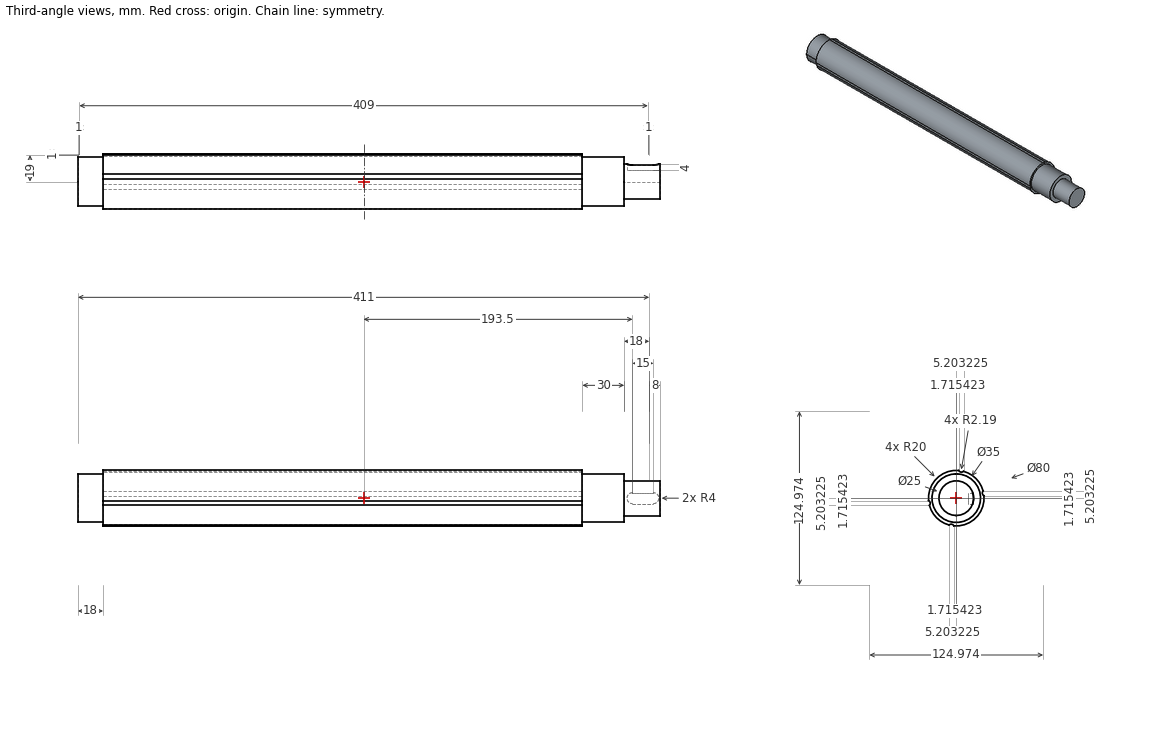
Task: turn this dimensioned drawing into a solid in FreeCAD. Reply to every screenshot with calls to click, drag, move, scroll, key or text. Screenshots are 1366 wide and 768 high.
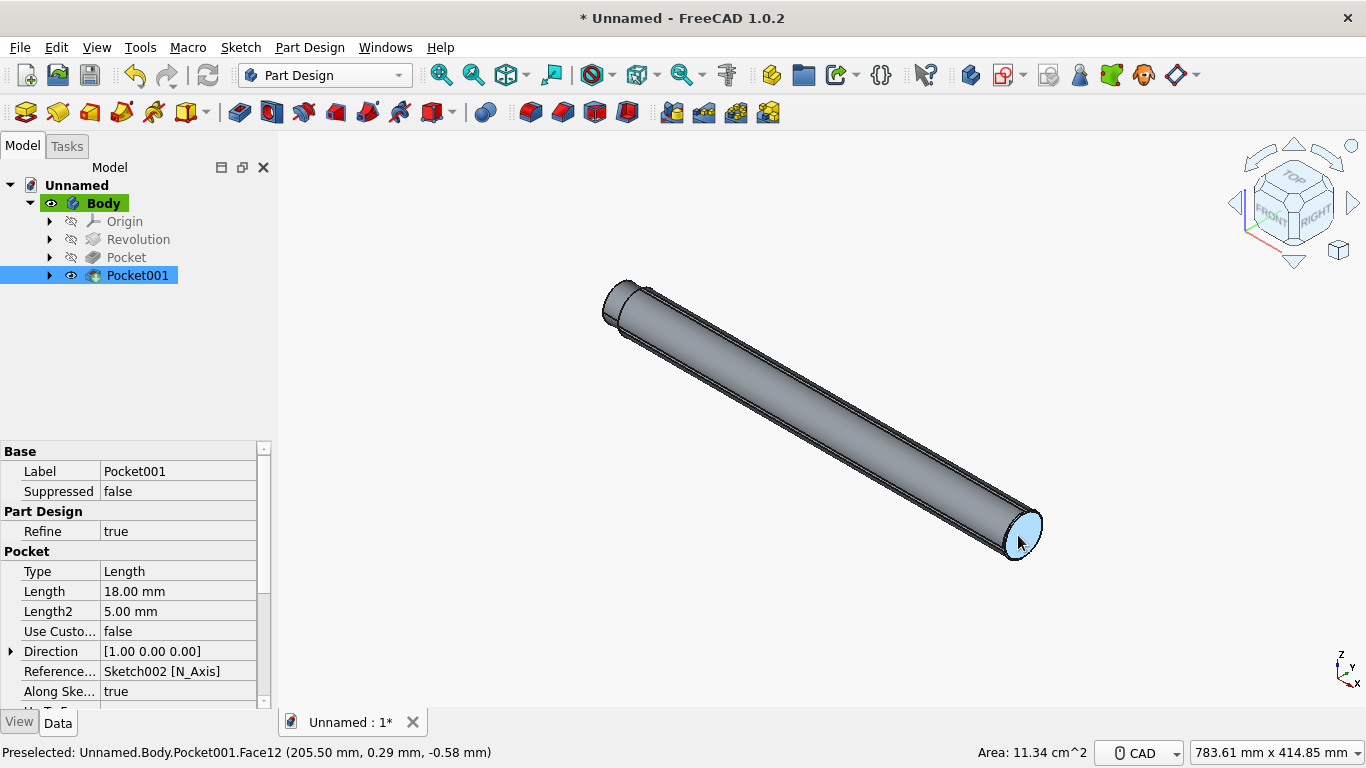
click(1004, 76)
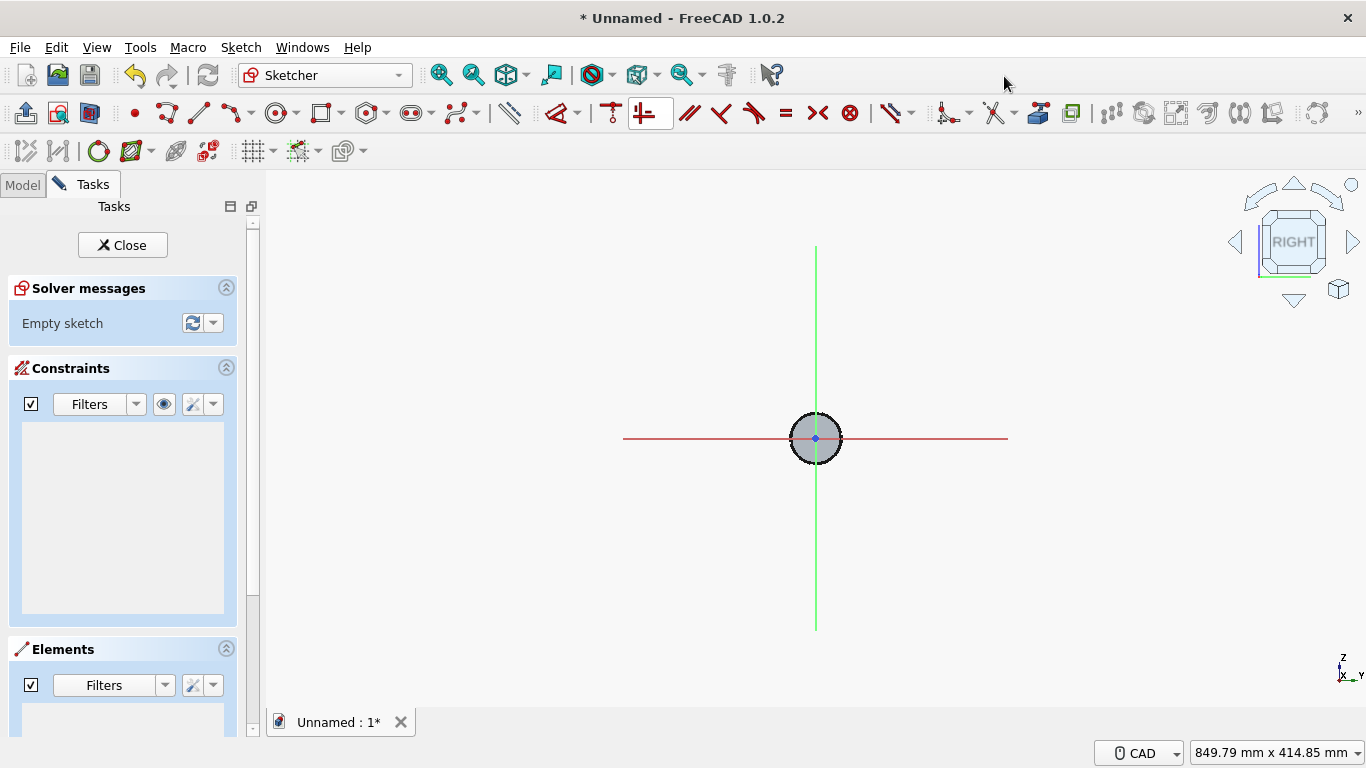
scroll(872, 438, up, 4)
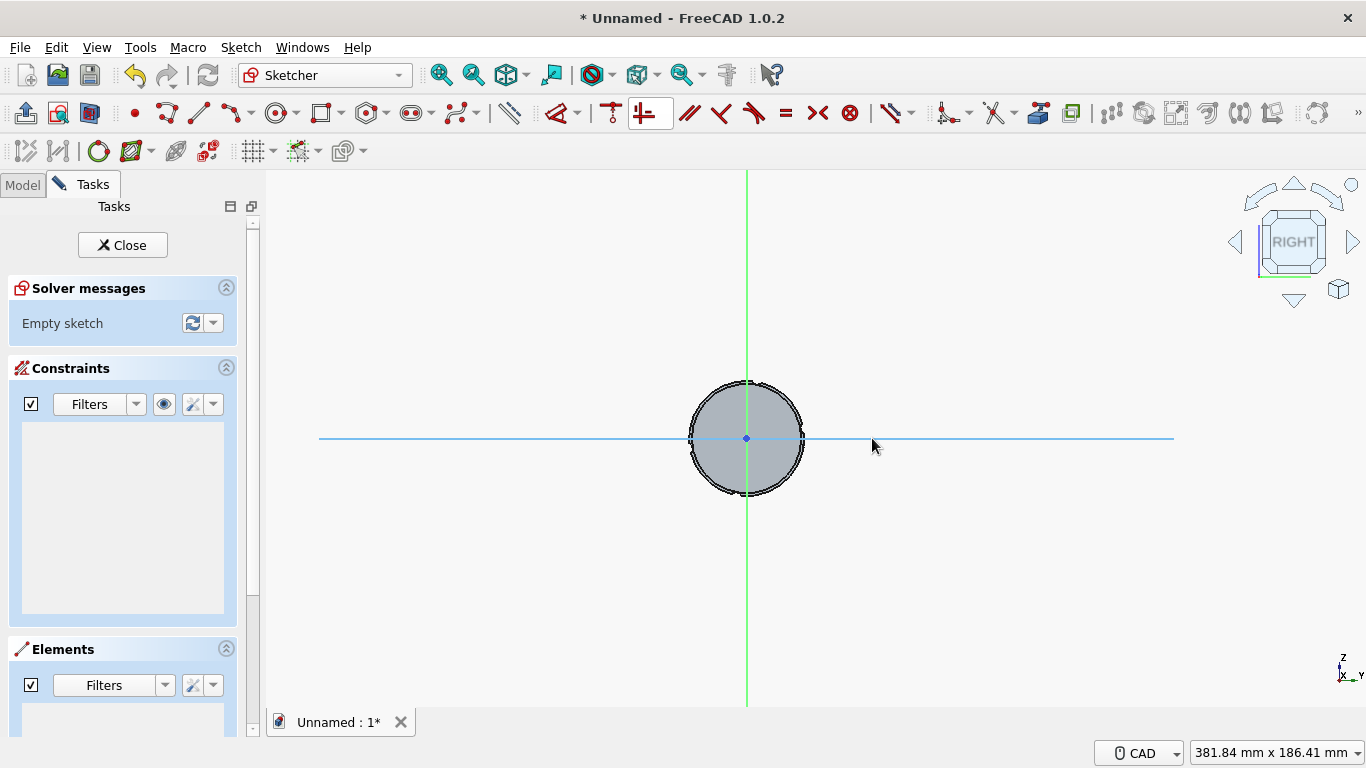
key(g)
key(v)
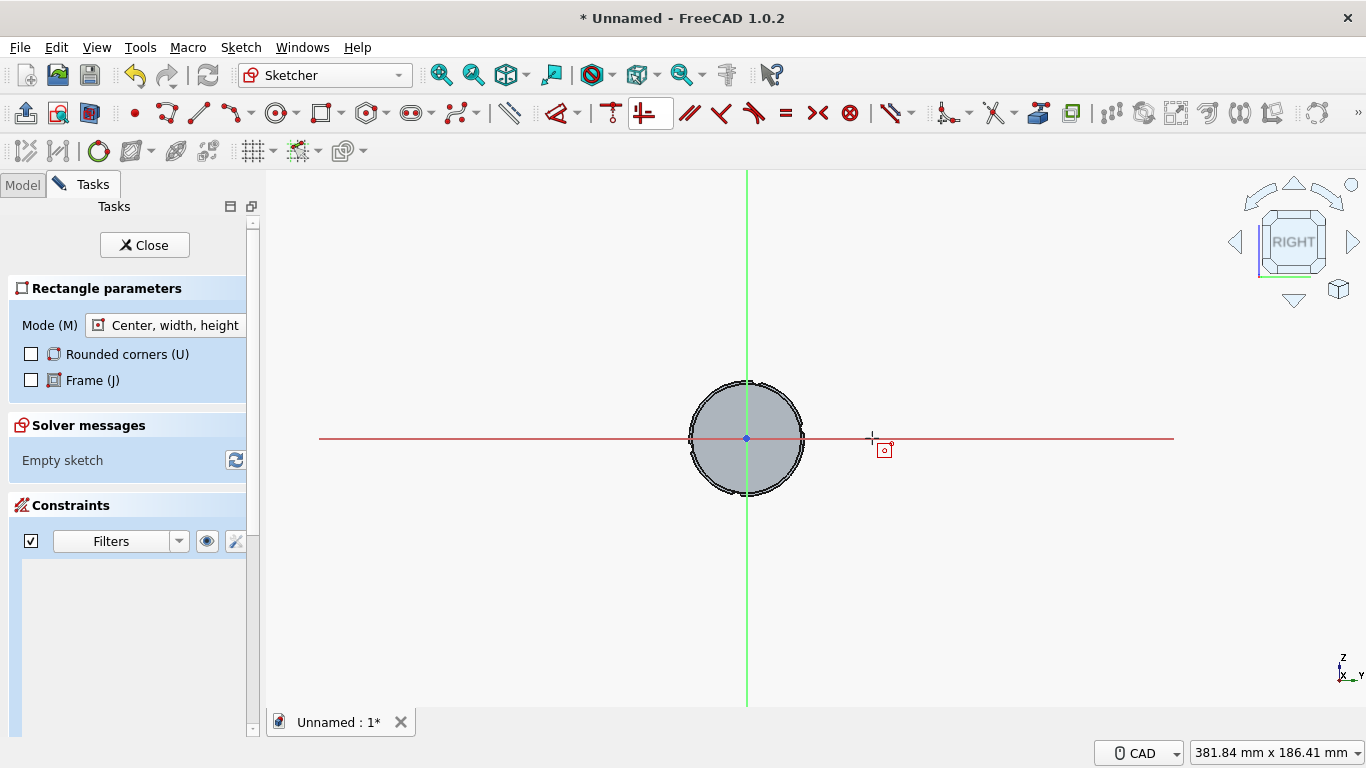
click(747, 438)
click(927, 258)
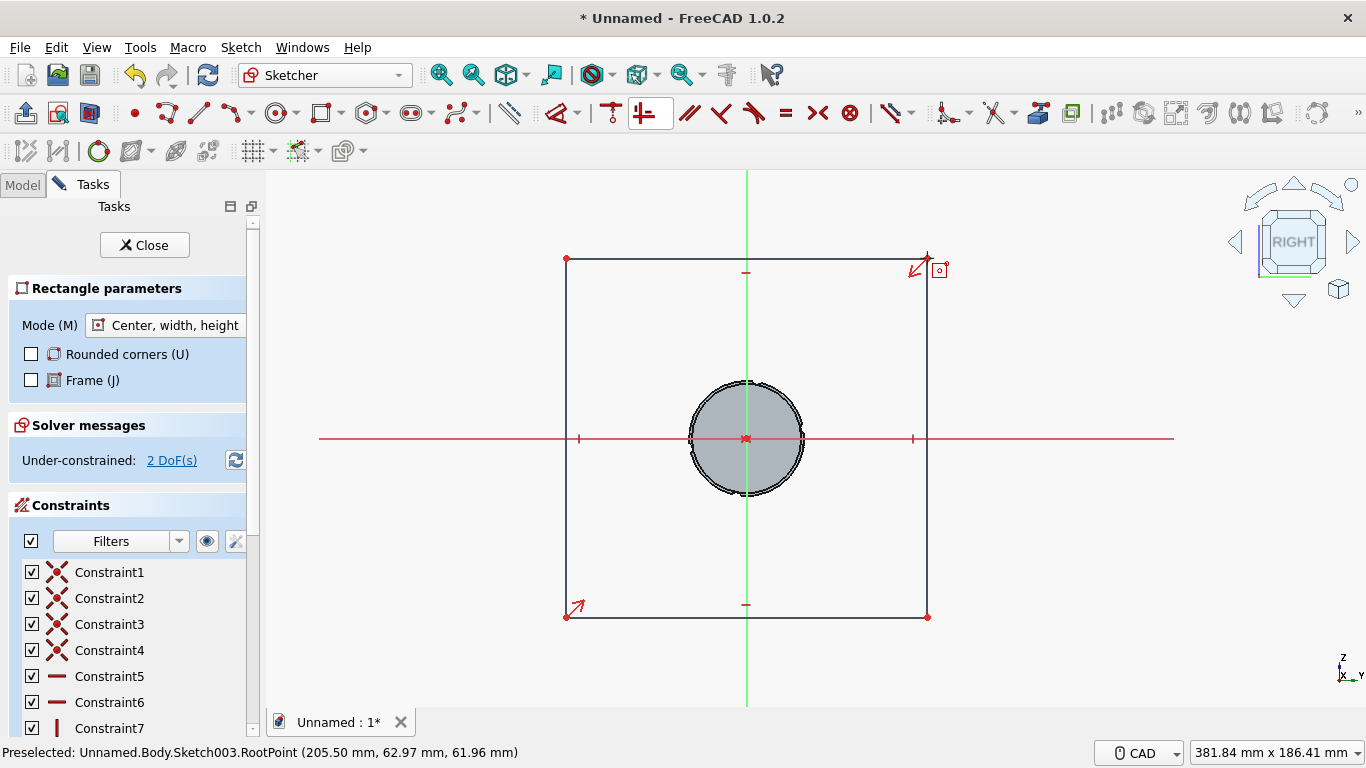
key(g)
key(c)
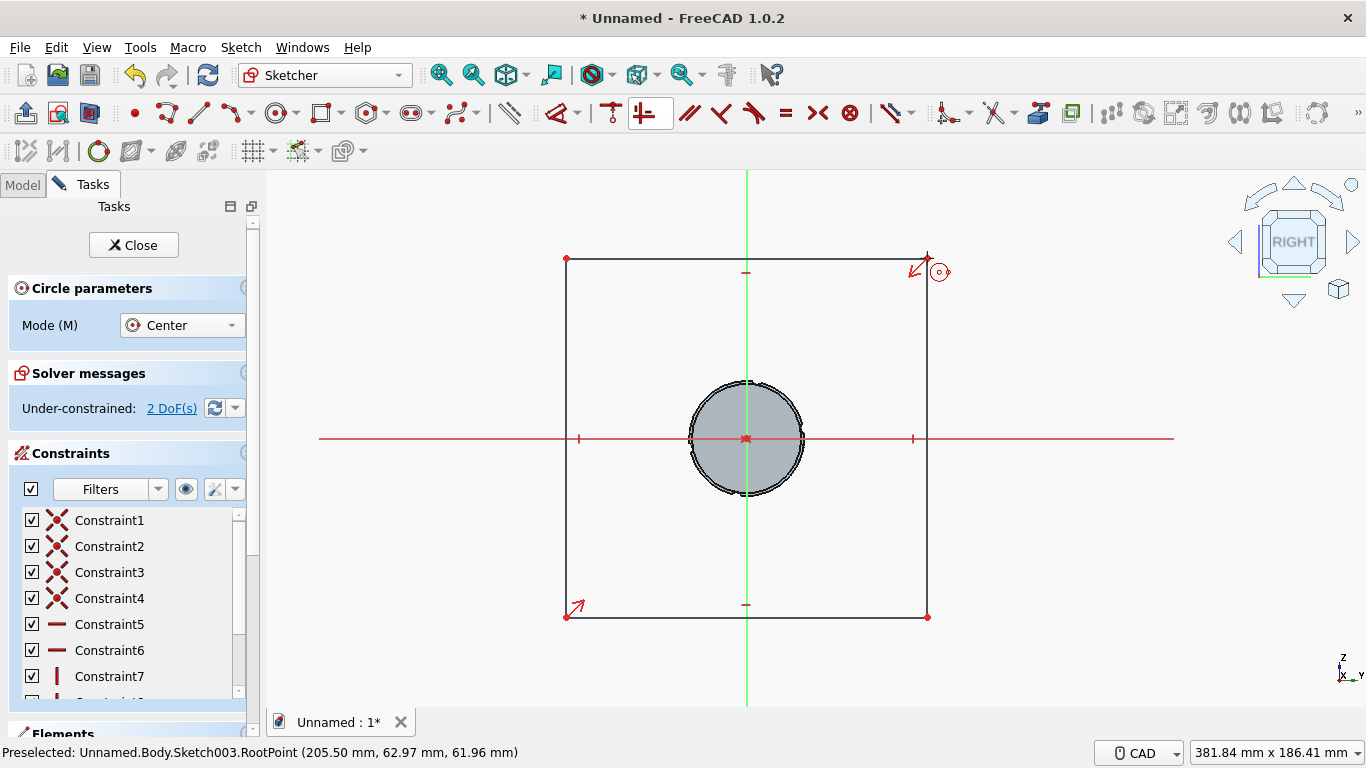
click(747, 438)
click(772, 413)
key(Escape)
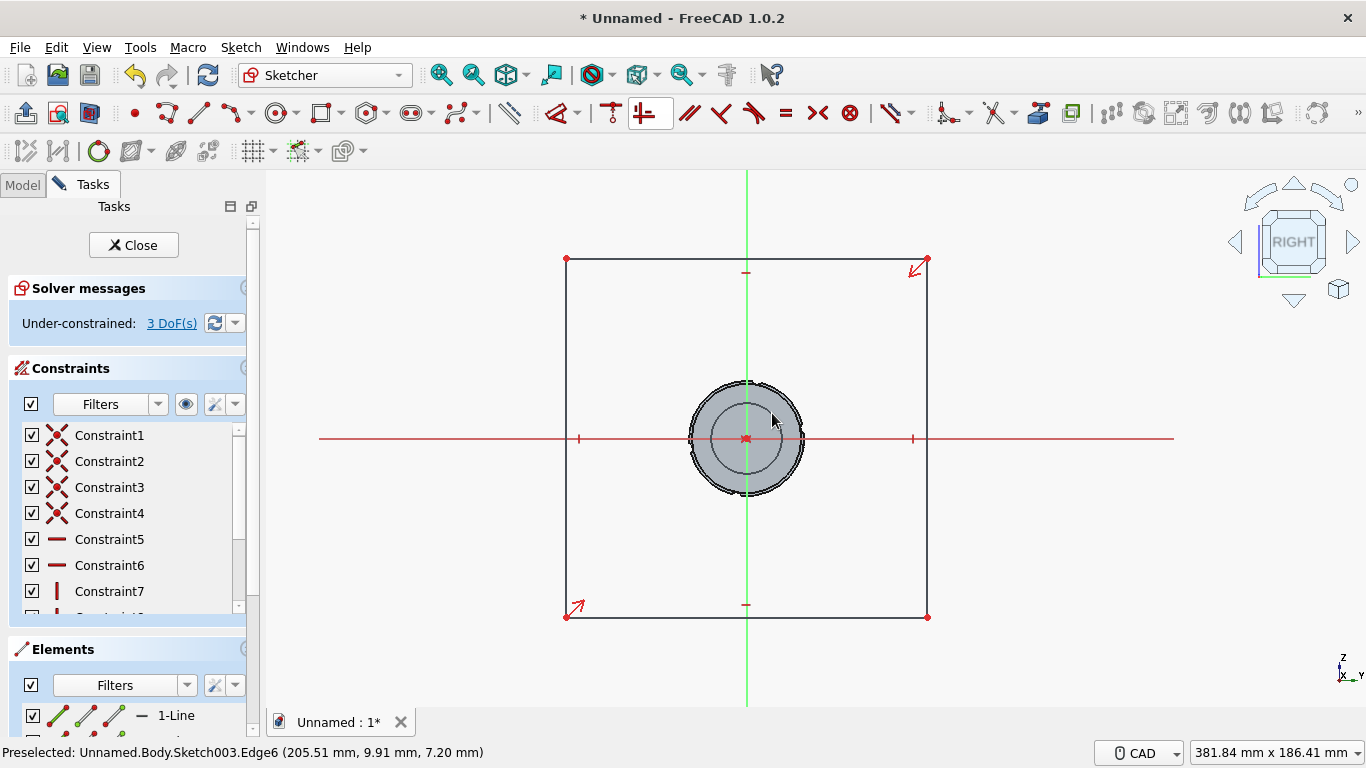
key(d)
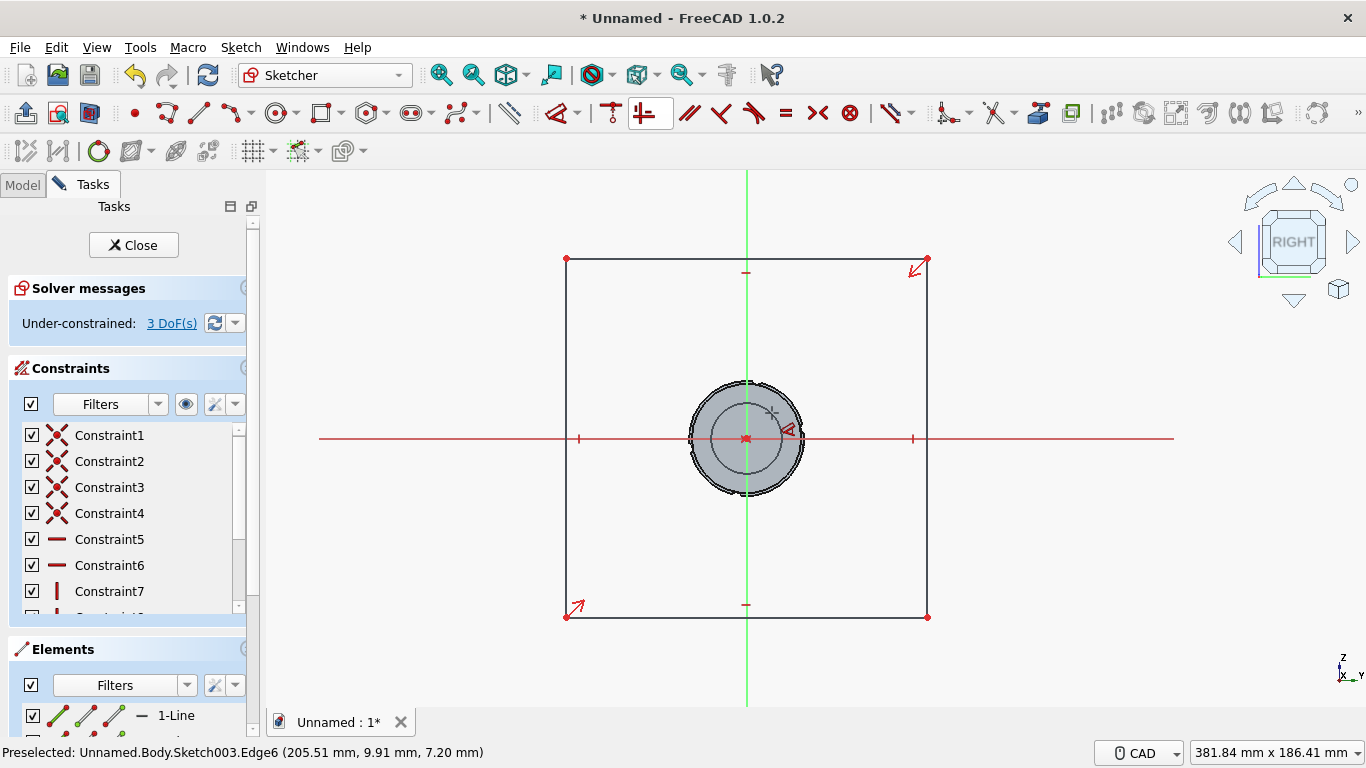
click(771, 413)
click(793, 390)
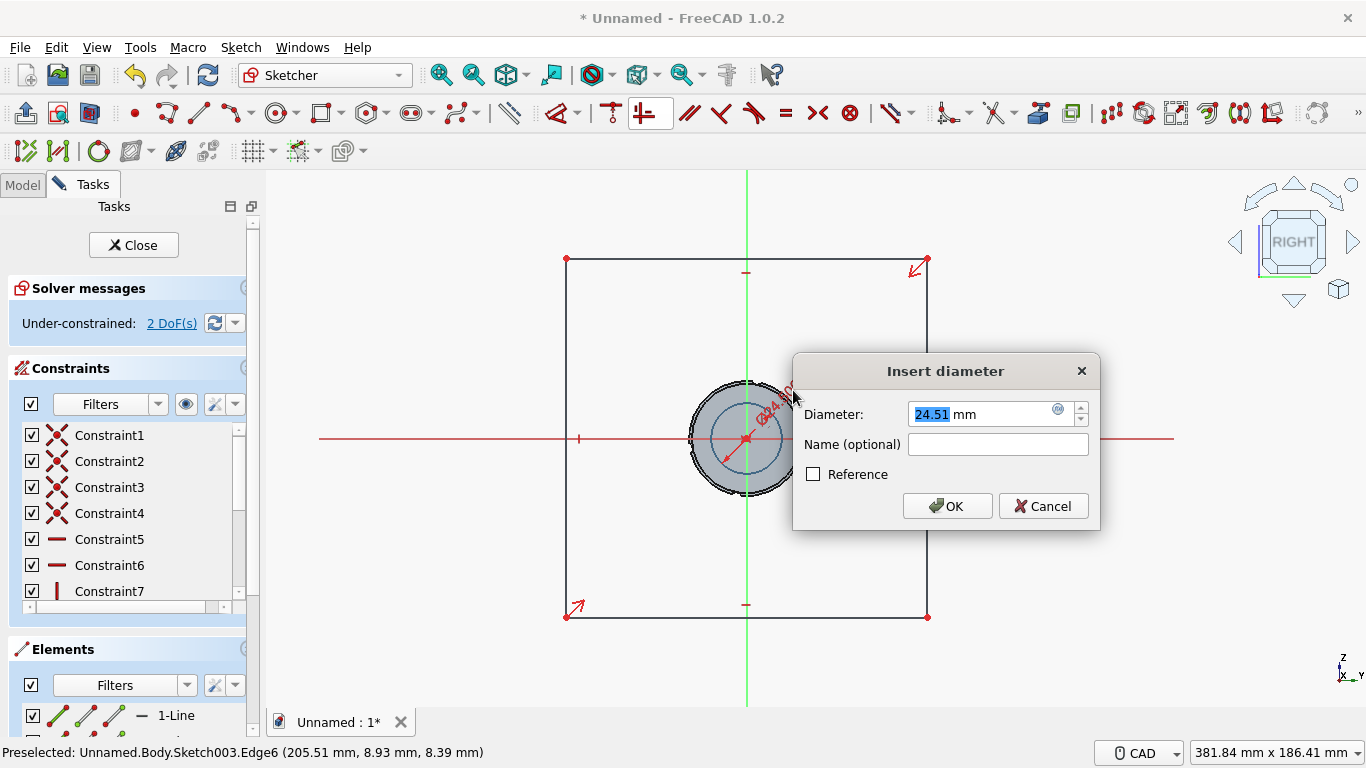
text(25)
key(Return)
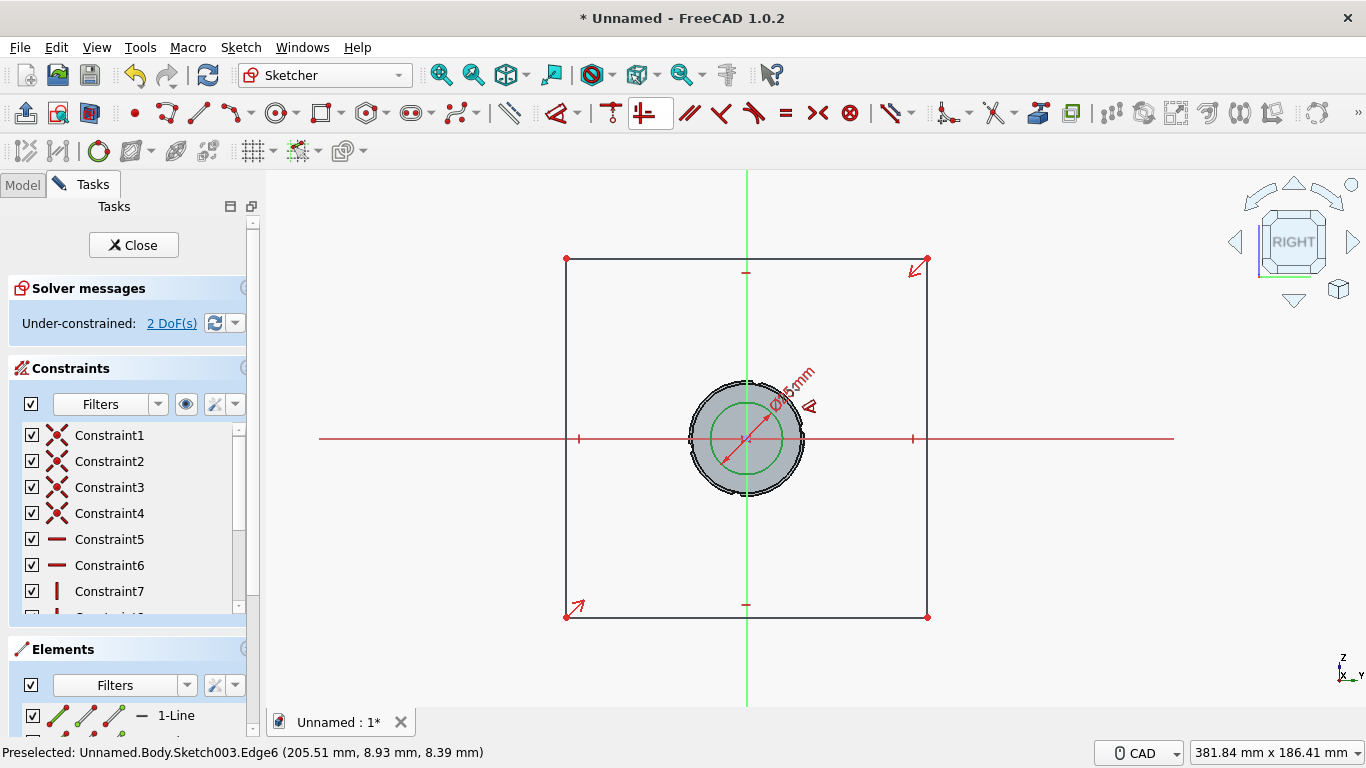
click(674, 618)
click(664, 652)